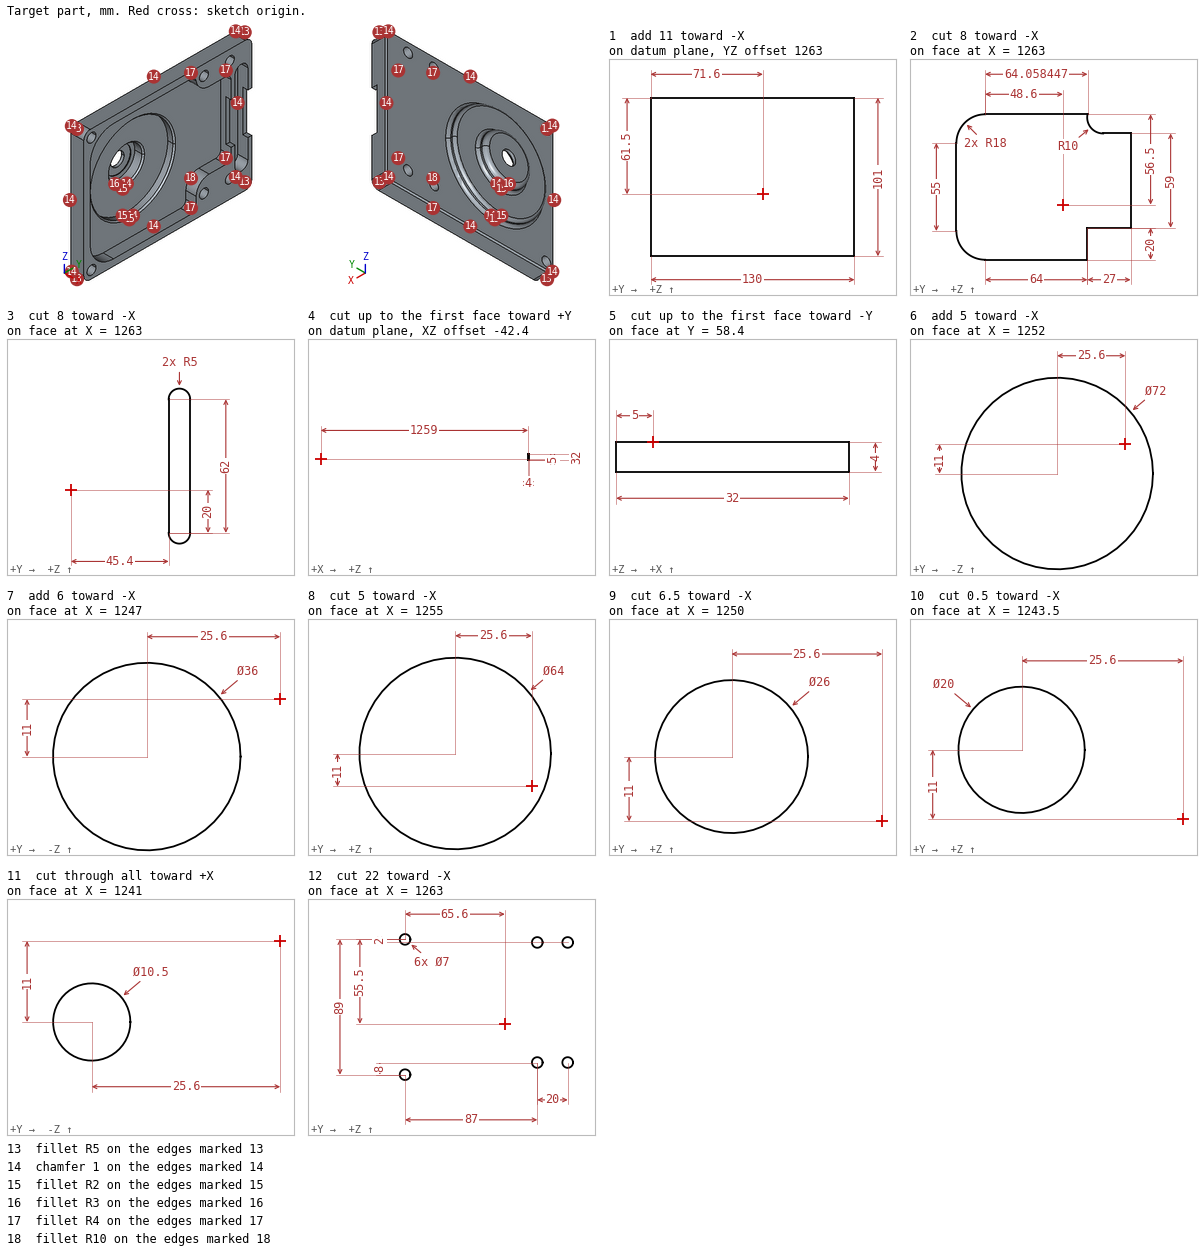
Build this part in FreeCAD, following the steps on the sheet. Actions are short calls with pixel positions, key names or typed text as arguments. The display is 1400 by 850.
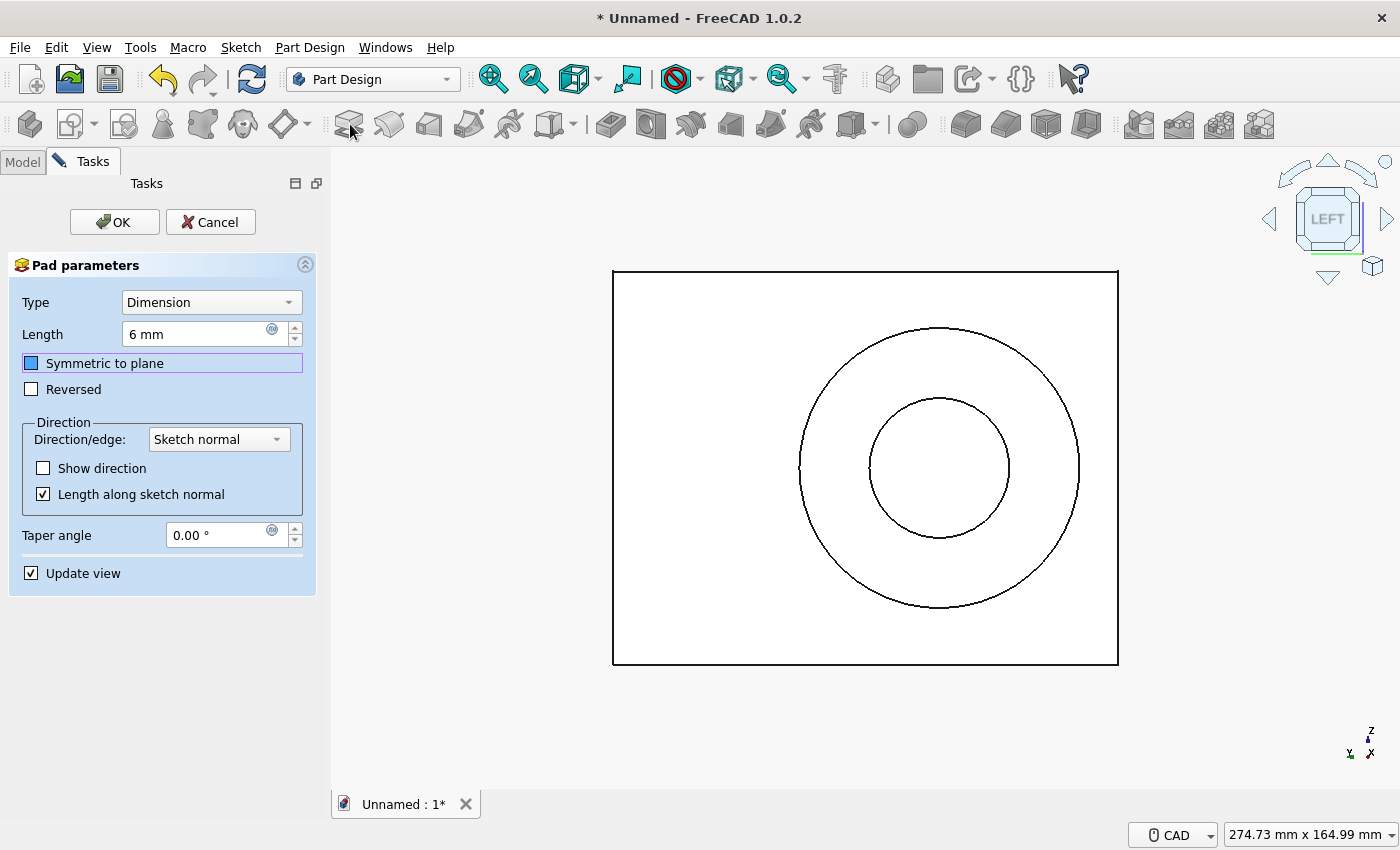
click(115, 222)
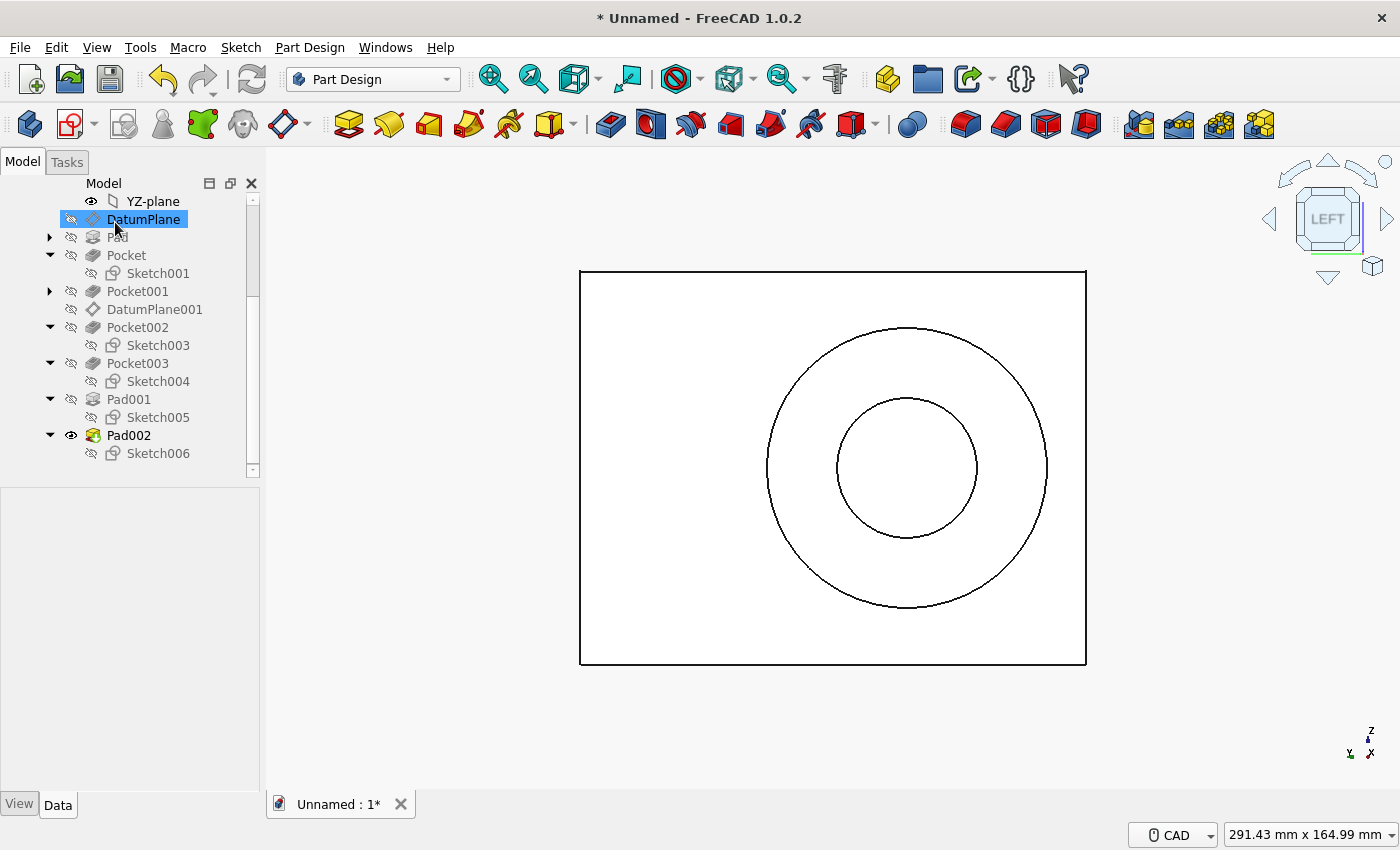
key(0)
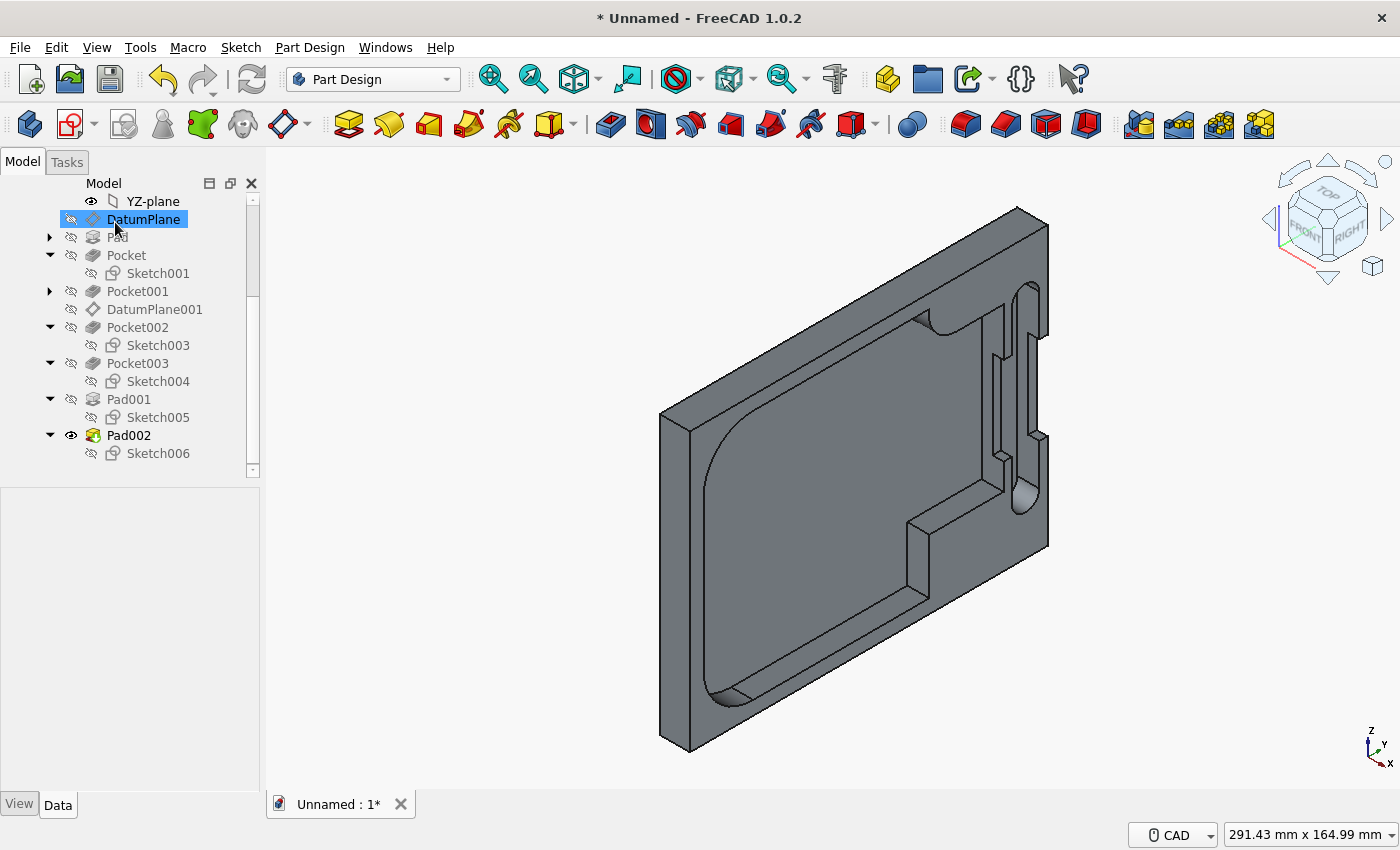
click(789, 508)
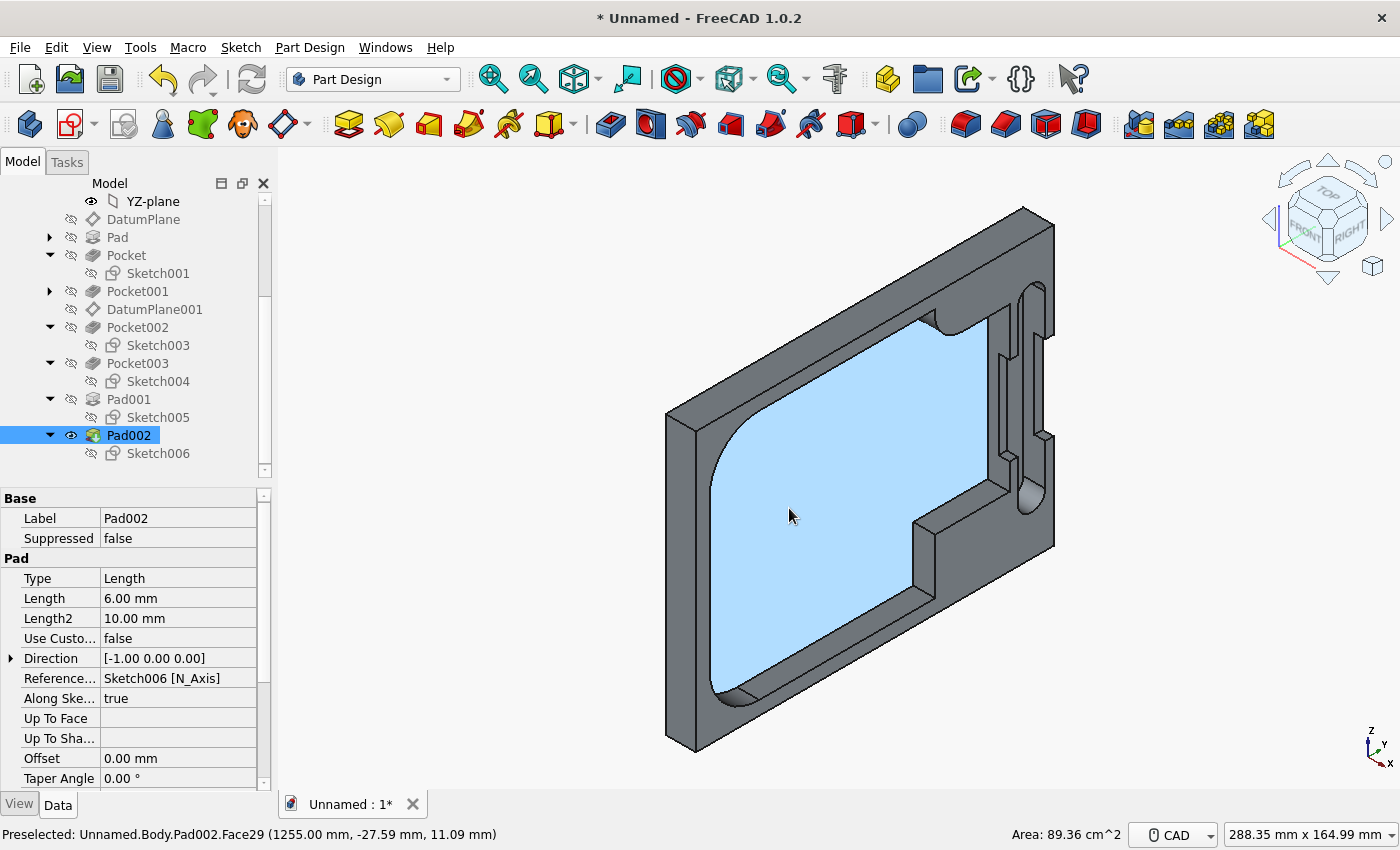
click(70, 124)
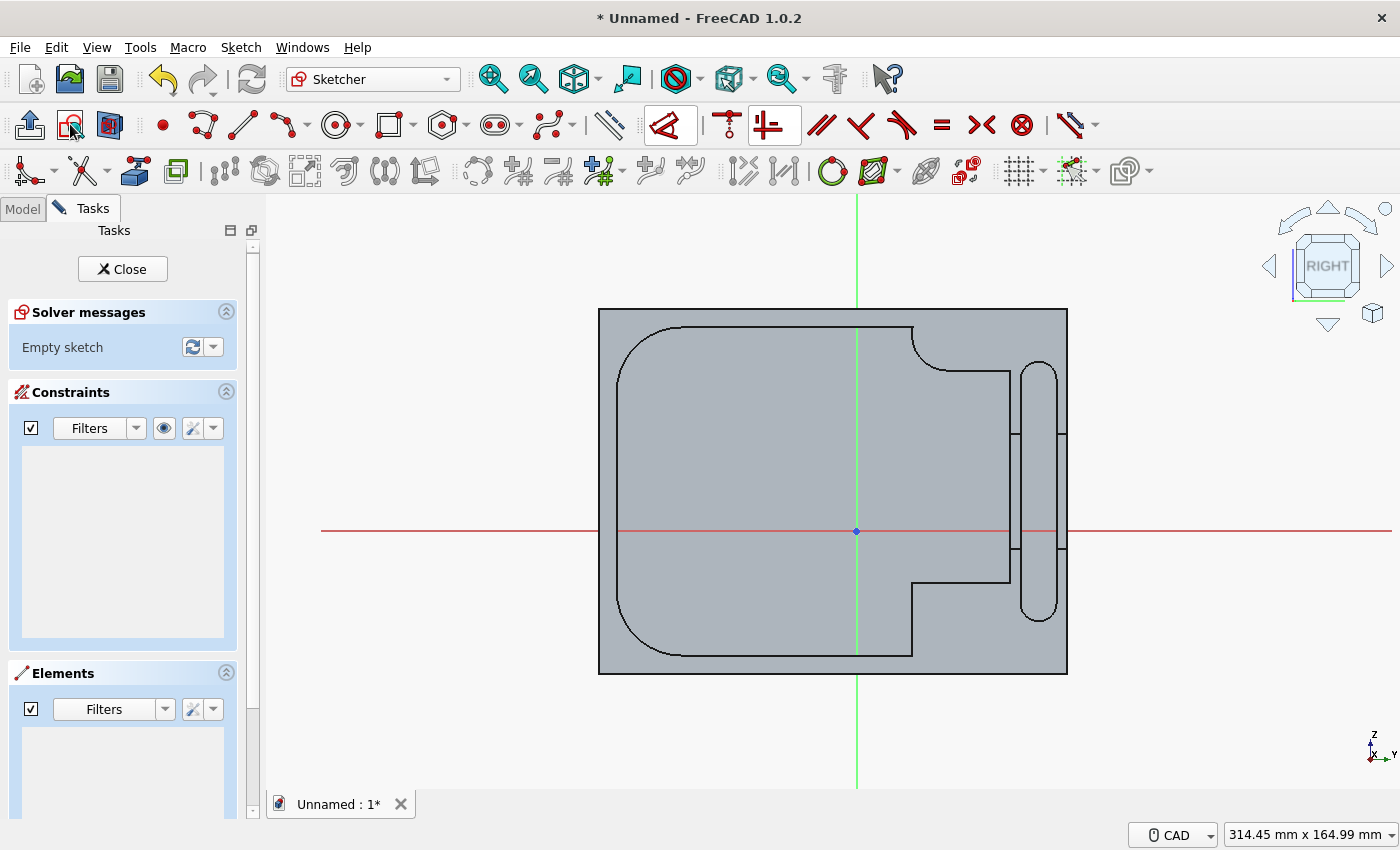
click(110, 126)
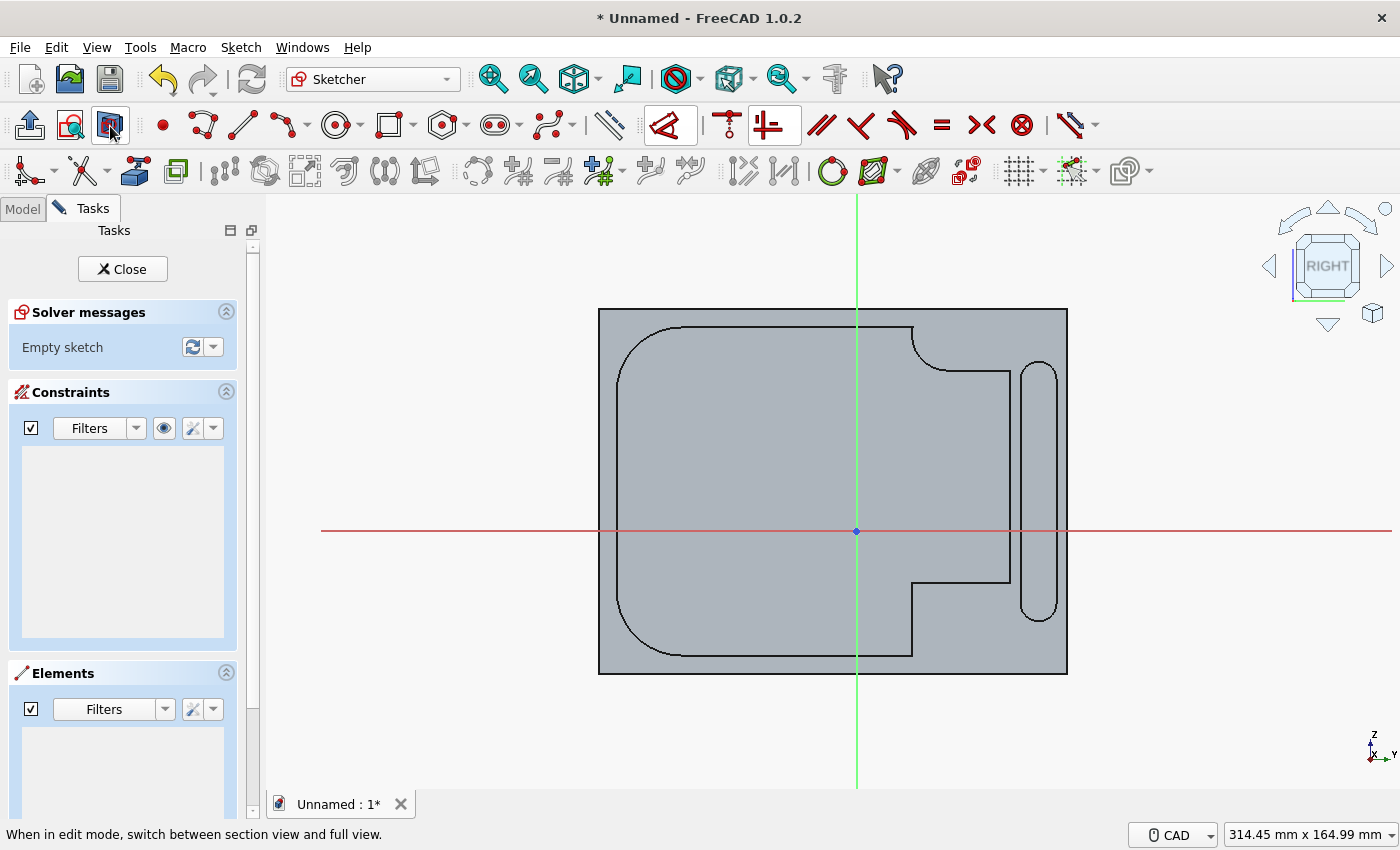
scroll(764, 492, up, 2)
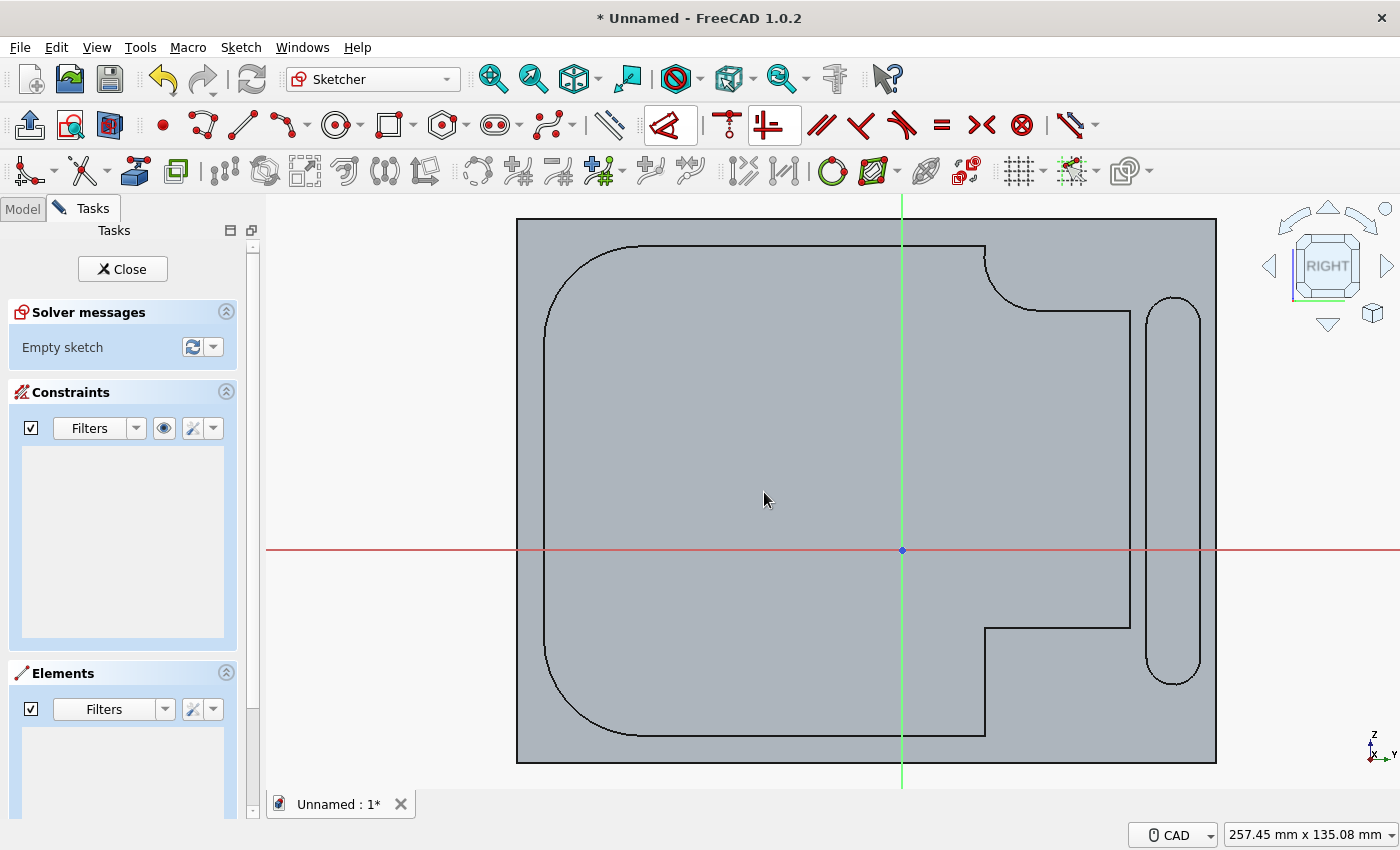
key(g)
key(c)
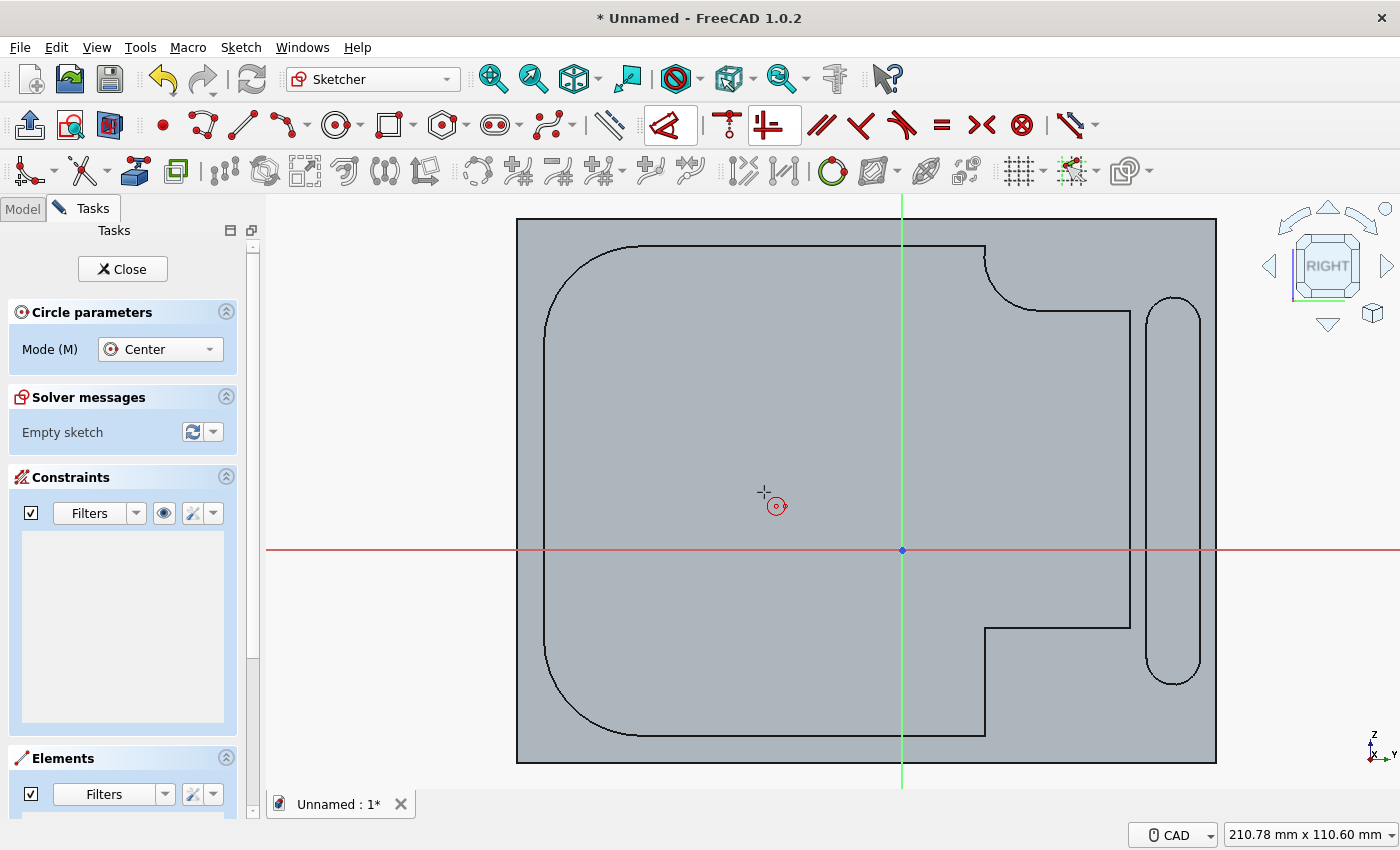
click(765, 491)
move(886, 369)